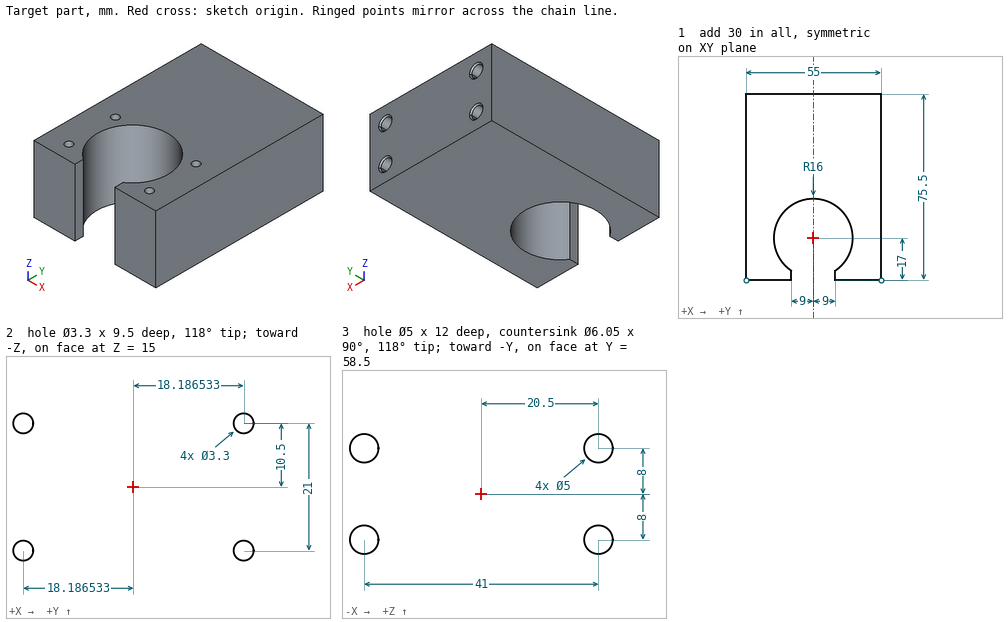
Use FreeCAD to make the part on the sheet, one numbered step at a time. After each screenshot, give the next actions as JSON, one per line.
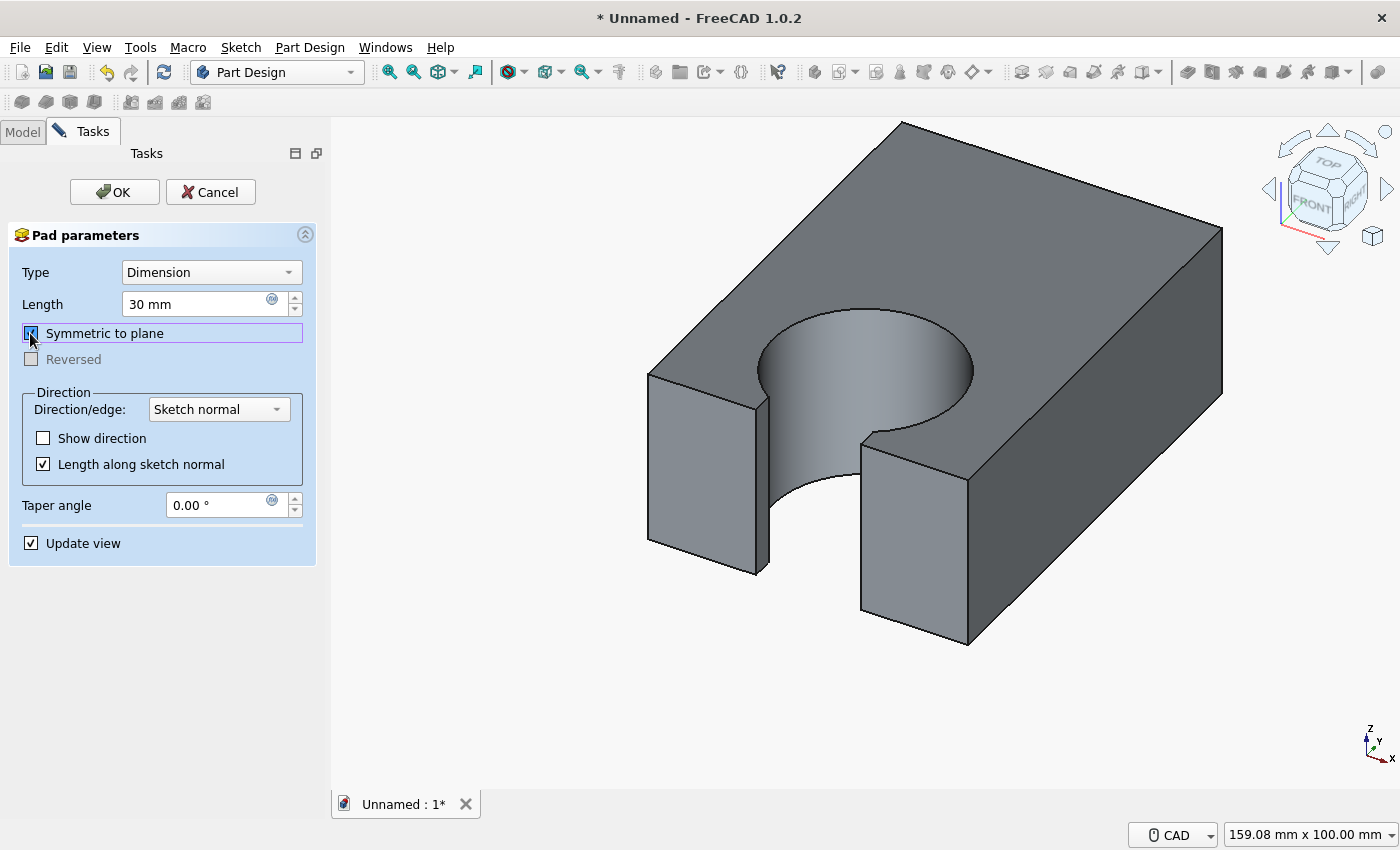
{"action": "left_click", "coordinate": [115, 192]}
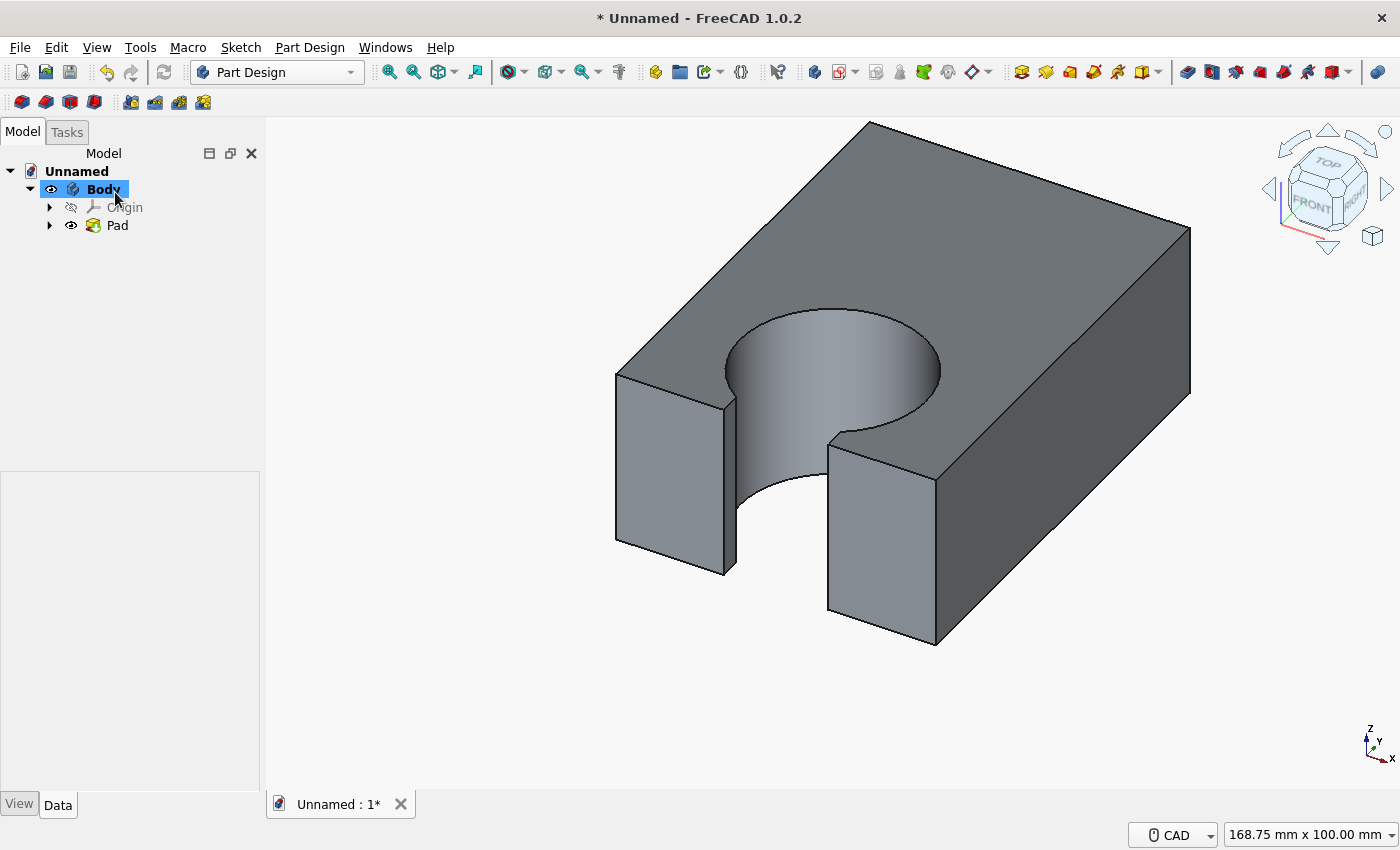
{"action": "left_click", "coordinate": [985, 279]}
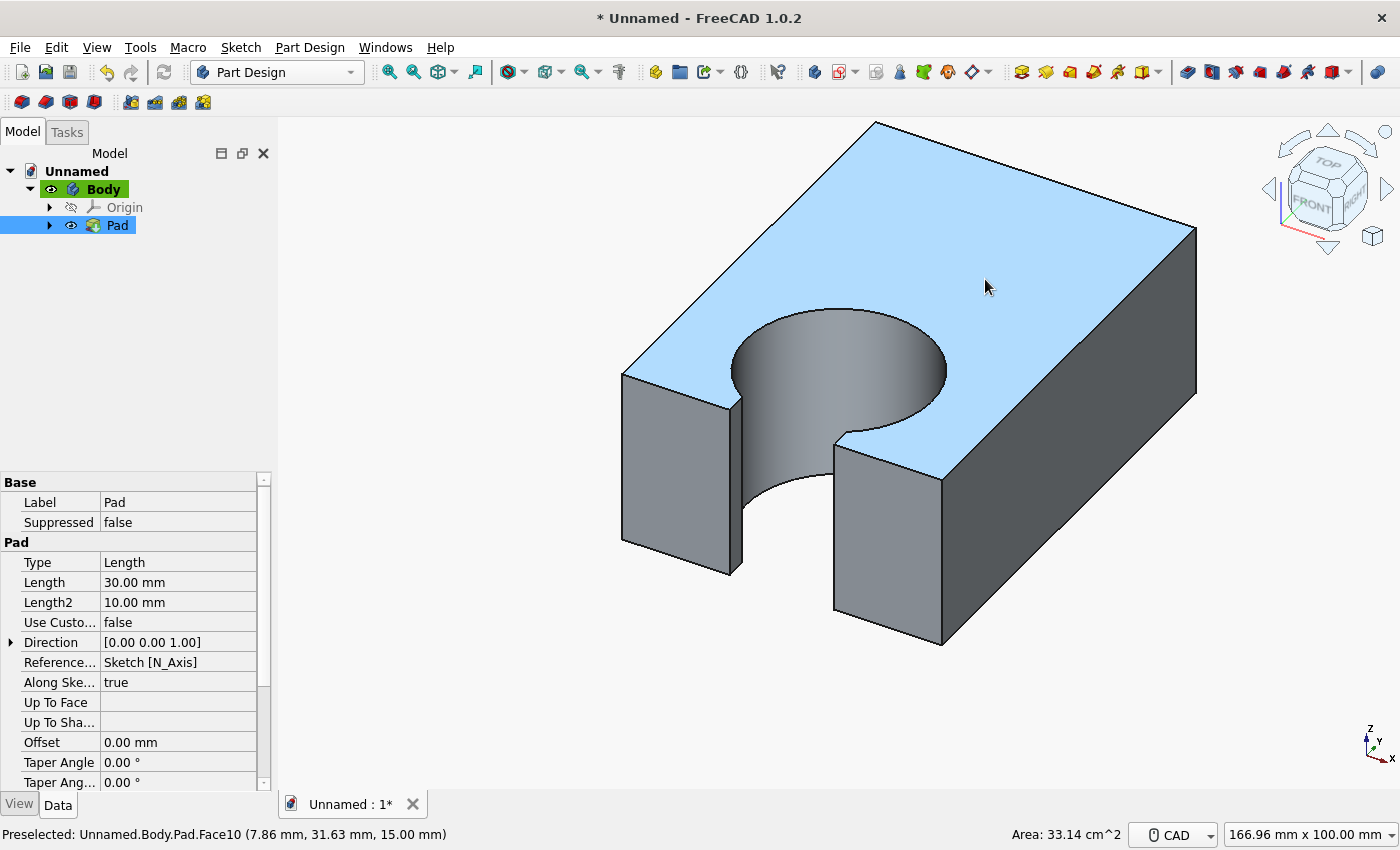
{"action": "left_click", "coordinate": [840, 72]}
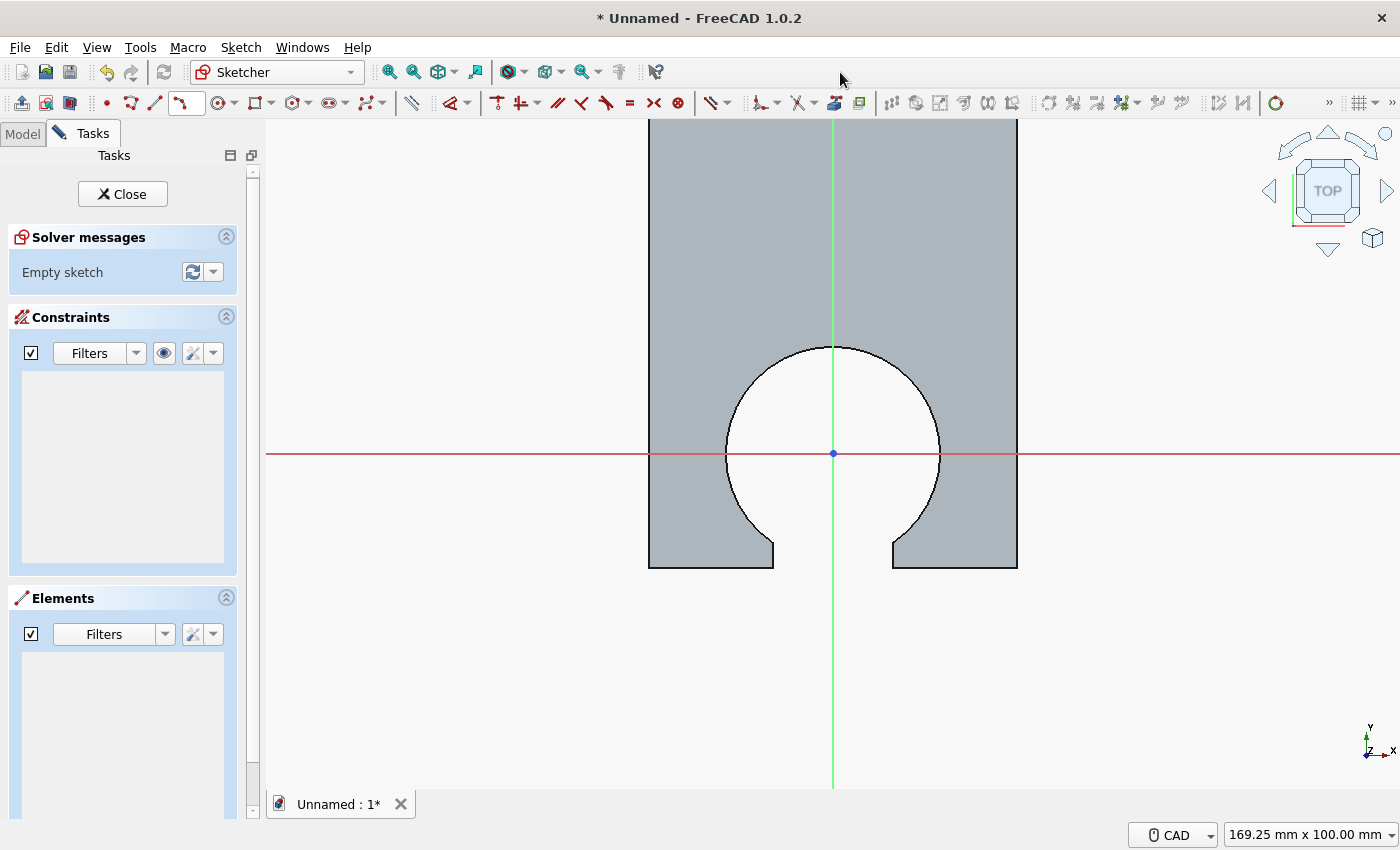
{"action": "scroll", "coordinate": [873, 454], "scroll_direction": "up", "scroll_amount": 5}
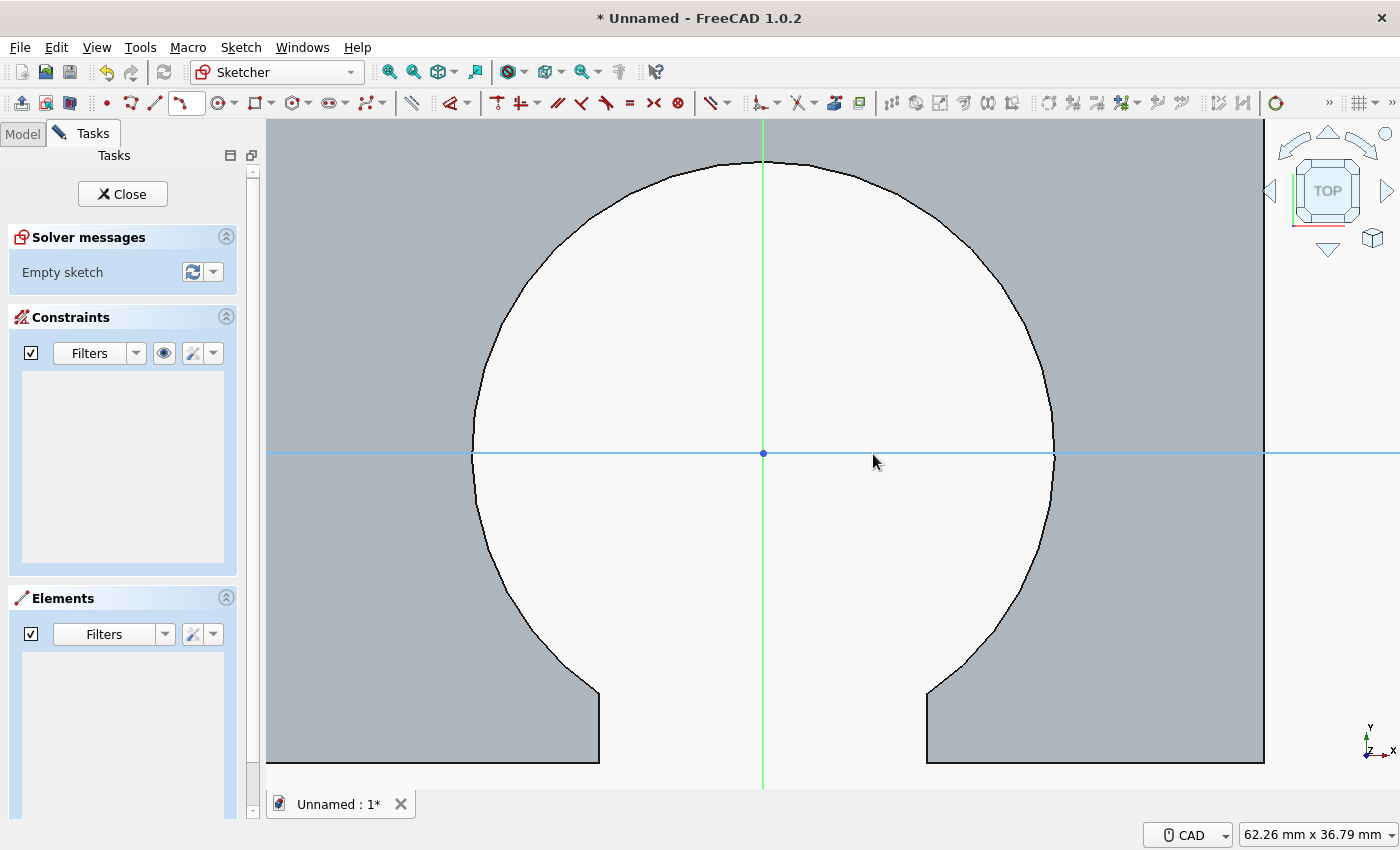
{"action": "left_click", "coordinate": [218, 104]}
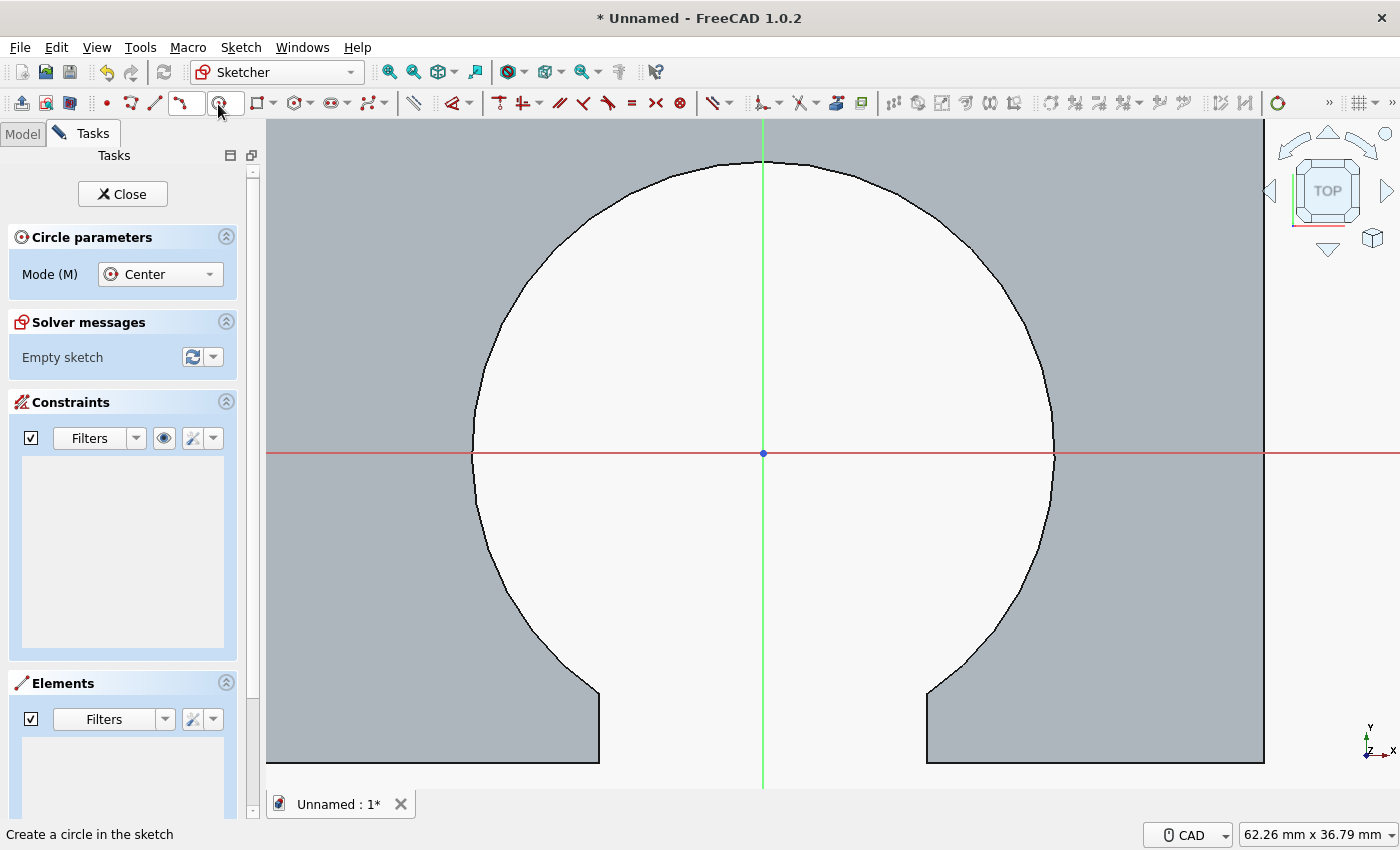
{"action": "left_click", "coordinate": [1095, 262]}
{"action": "left_click", "coordinate": [1116, 241]}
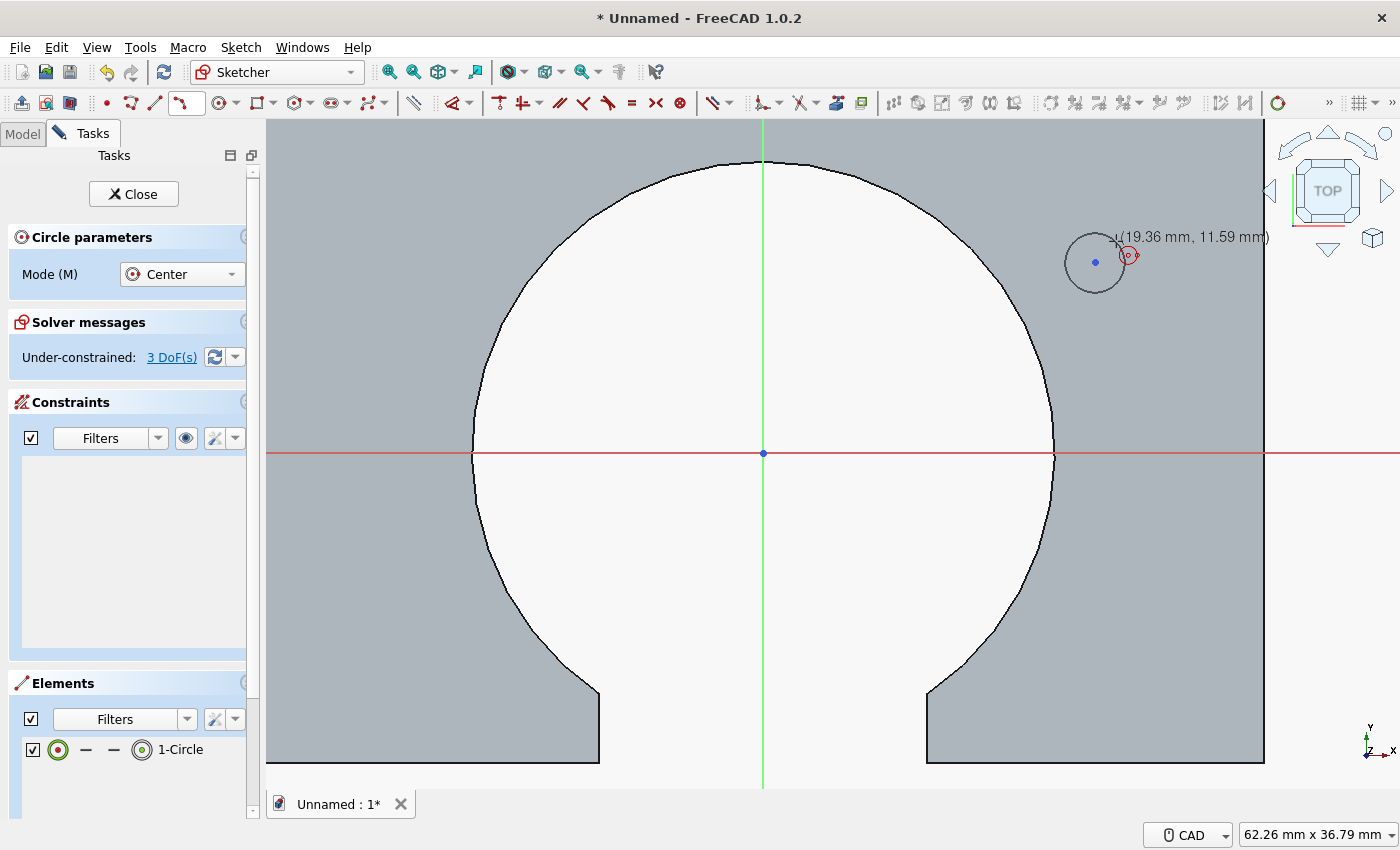
{"action": "left_click", "coordinate": [1095, 644]}
{"action": "left_click", "coordinate": [1116, 623]}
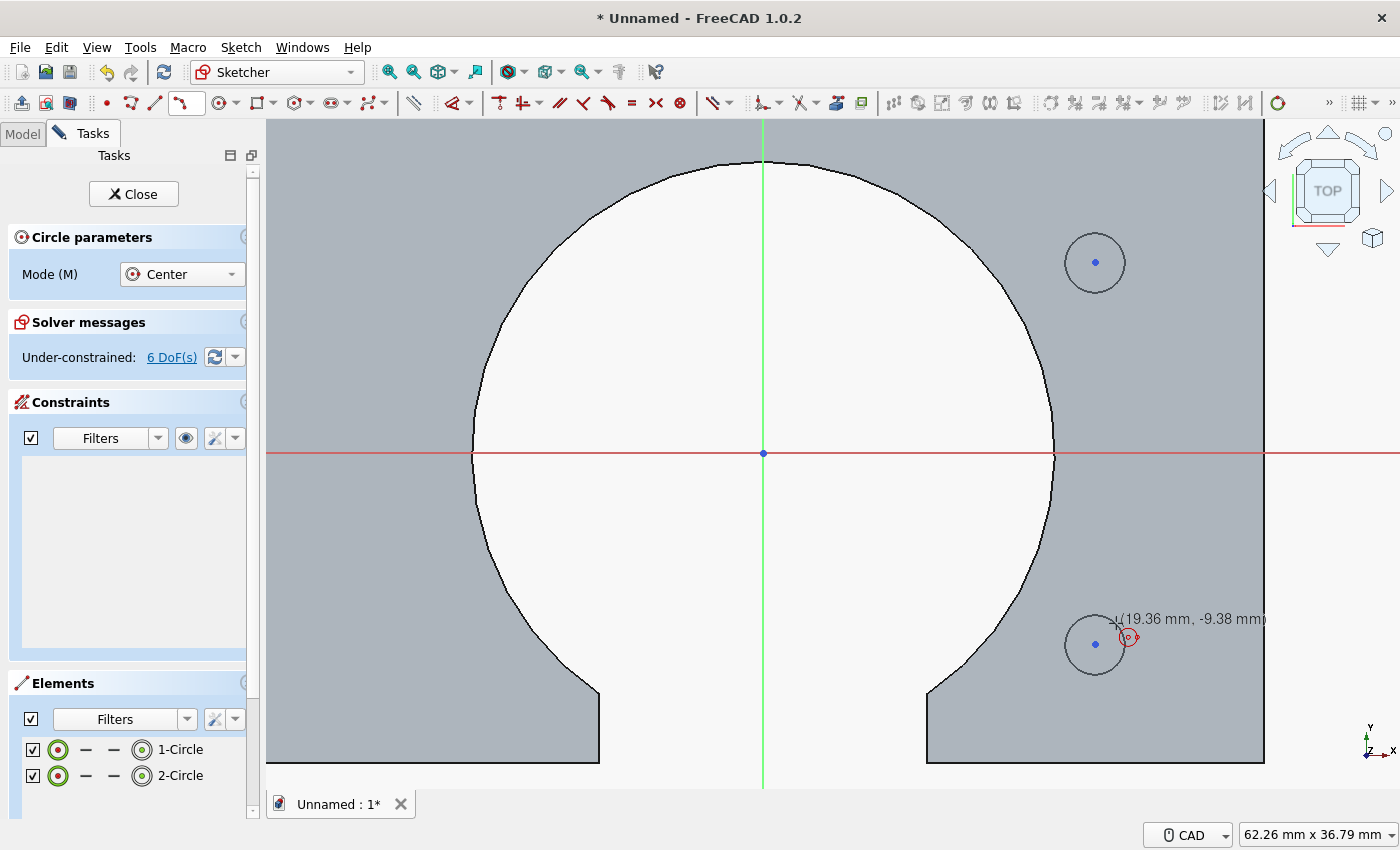
{"action": "left_click", "coordinate": [432, 644]}
{"action": "left_click", "coordinate": [453, 623]}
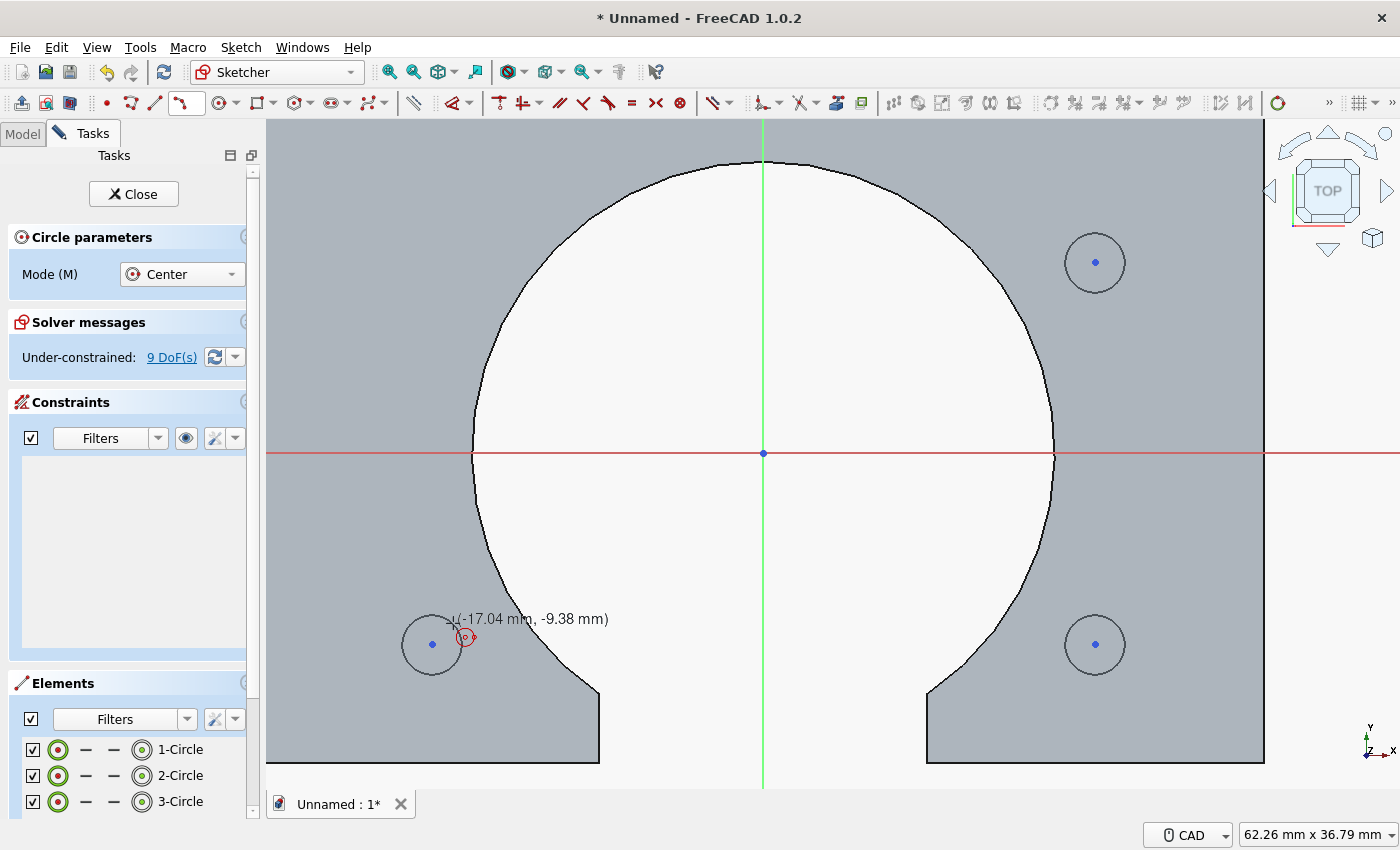
{"action": "left_click", "coordinate": [432, 262]}
{"action": "left_click", "coordinate": [453, 241]}
{"action": "key", "text": "Escape"}